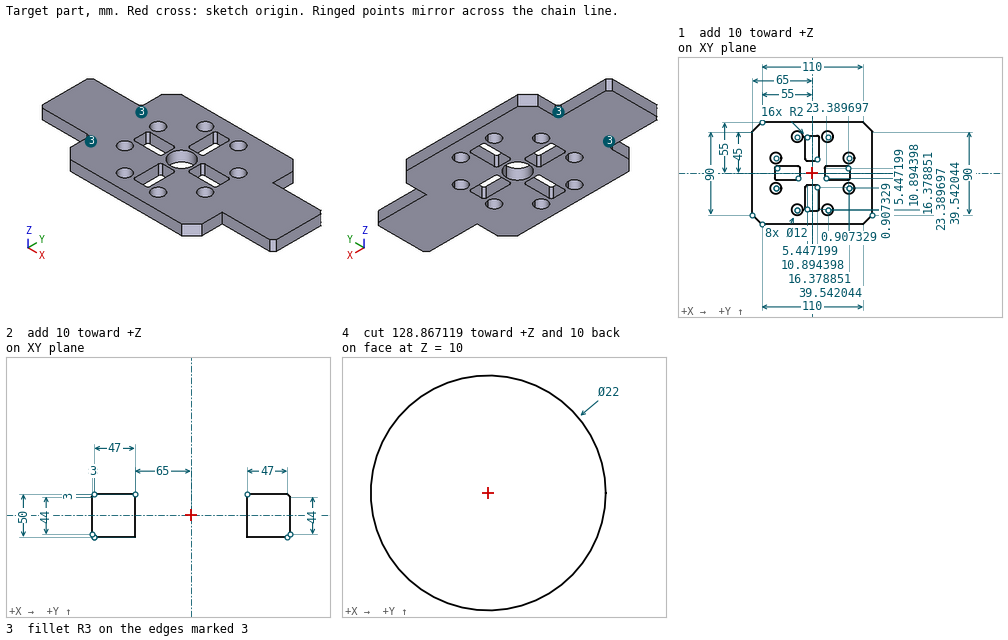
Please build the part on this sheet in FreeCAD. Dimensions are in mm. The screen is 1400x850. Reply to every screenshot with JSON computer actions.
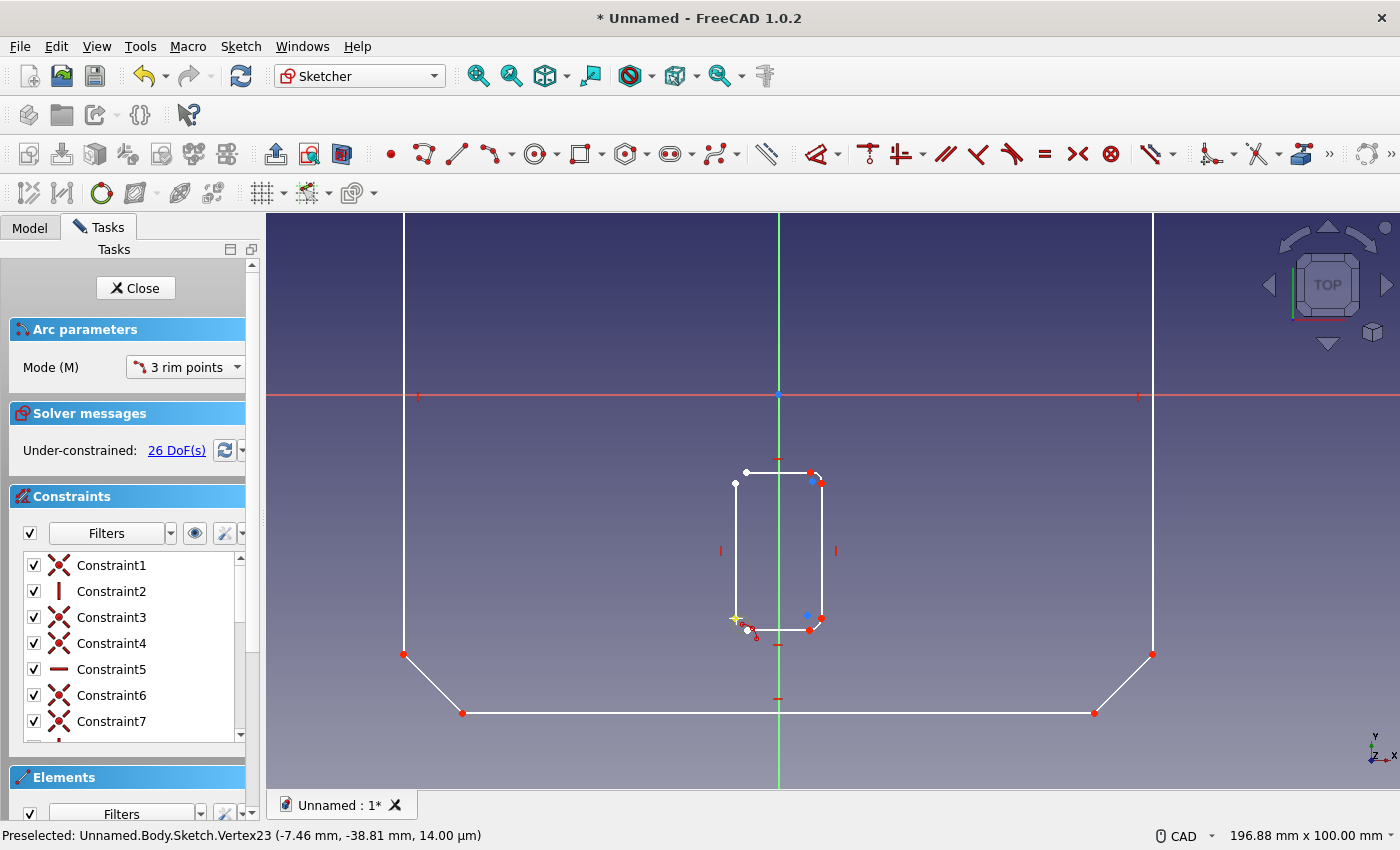
{"action": "scroll", "coordinate": [739, 625], "scroll_direction": "up", "scroll_amount": 8}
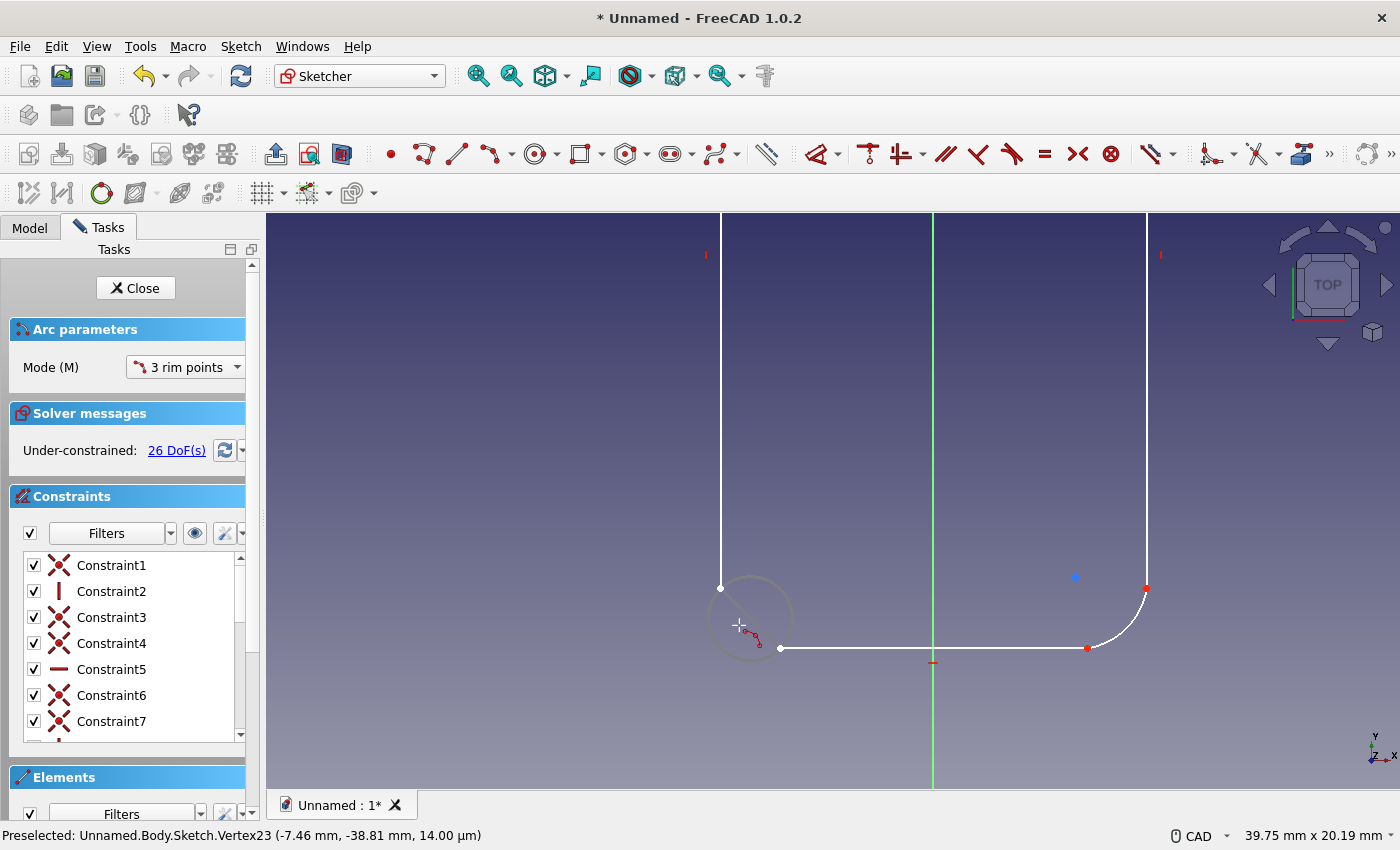
{"action": "left_click", "coordinate": [738, 624]}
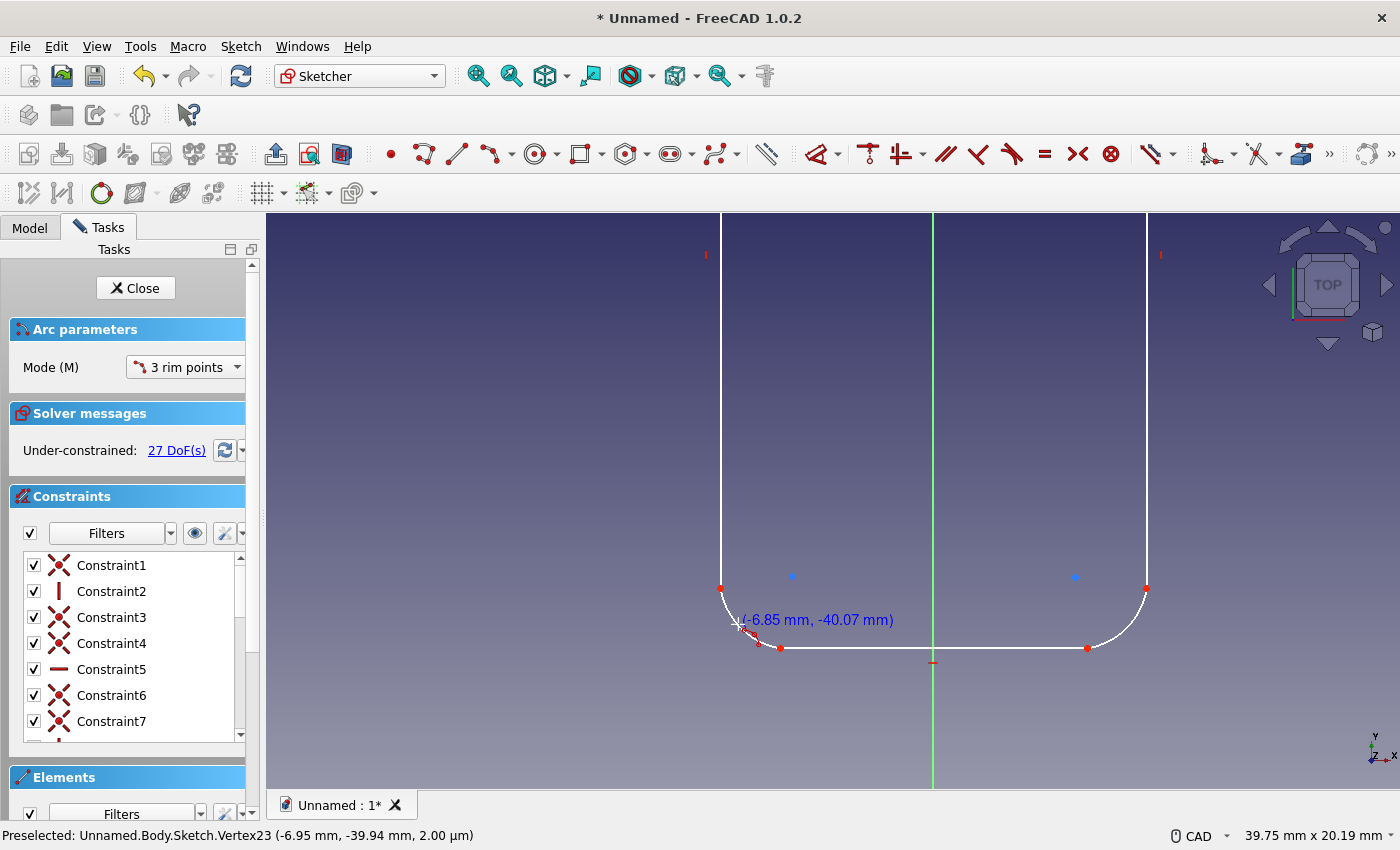
{"action": "scroll", "coordinate": [743, 628], "scroll_direction": "down", "scroll_amount": 11}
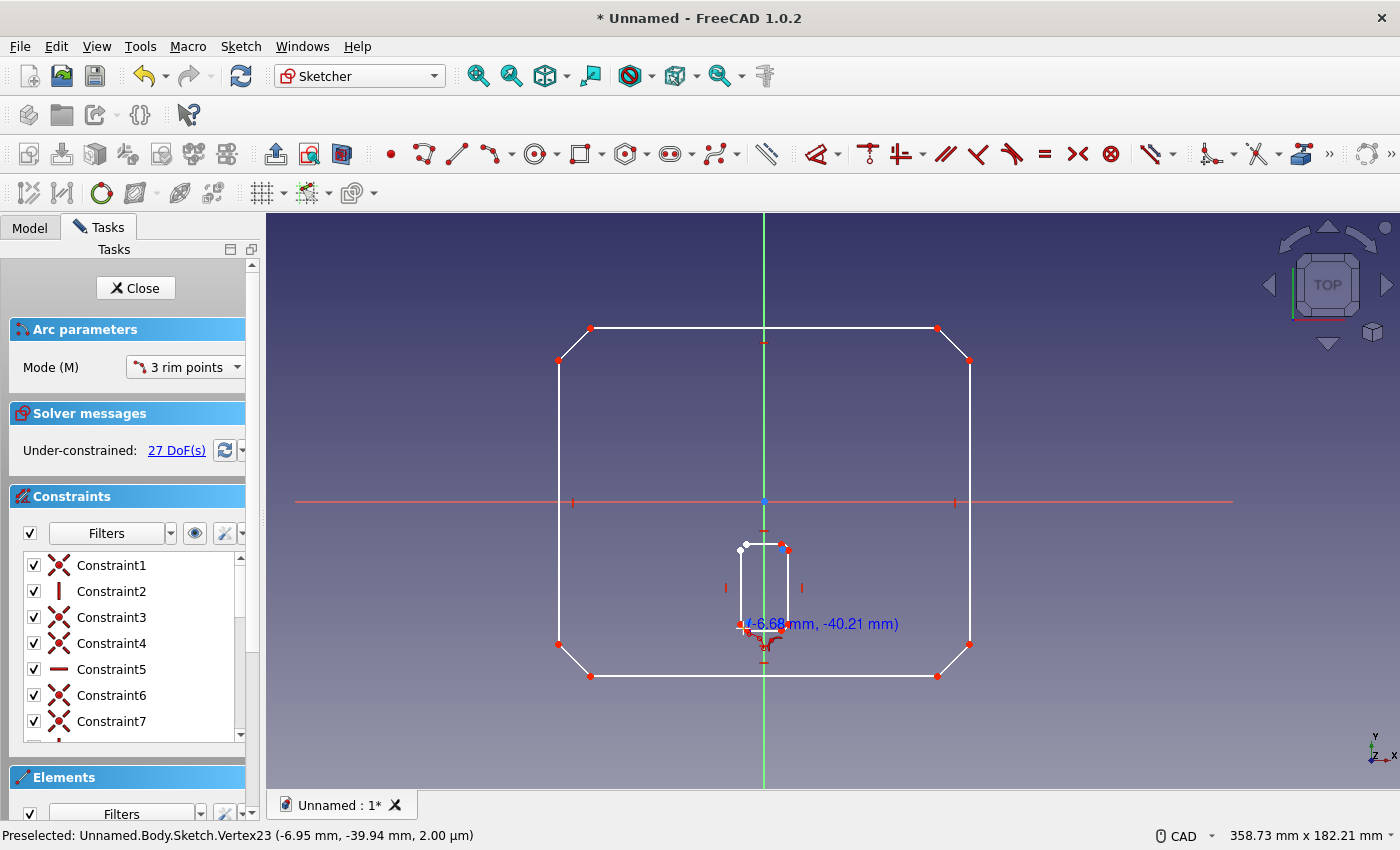
{"action": "scroll", "coordinate": [741, 550], "scroll_direction": "up", "scroll_amount": 3}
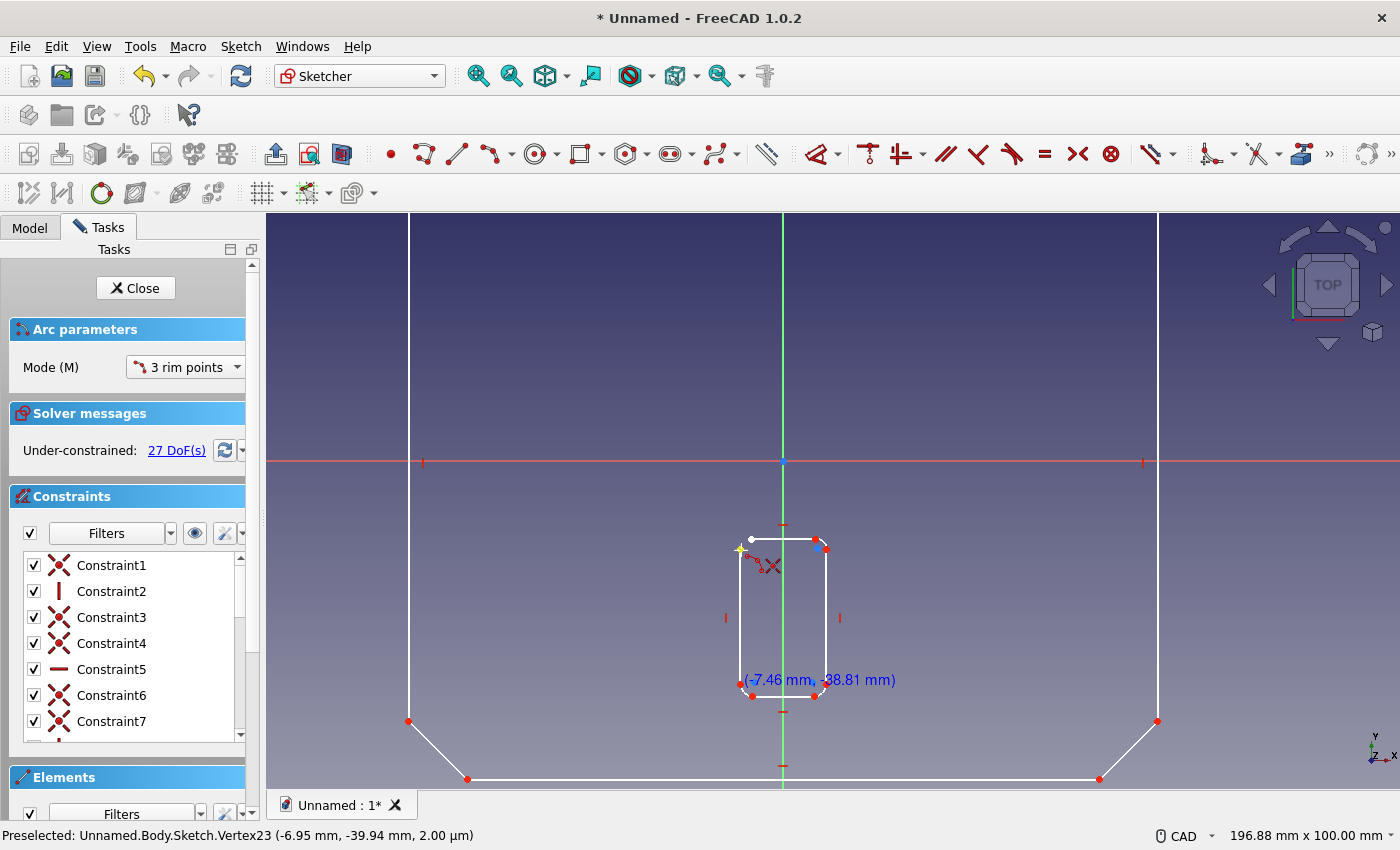
{"action": "left_click", "coordinate": [740, 550]}
{"action": "left_click", "coordinate": [751, 539]}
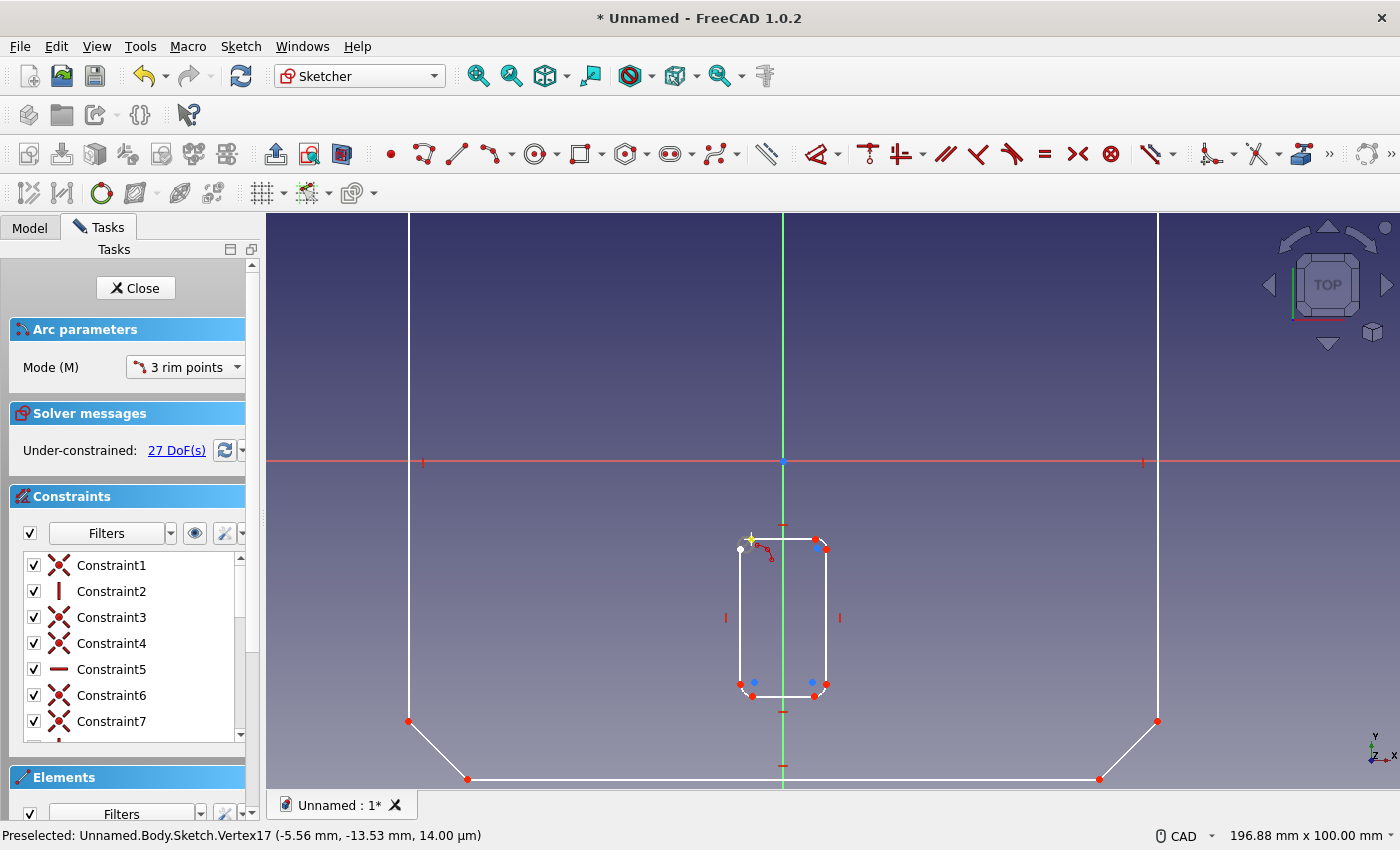
{"action": "scroll", "coordinate": [744, 541], "scroll_direction": "up", "scroll_amount": 8}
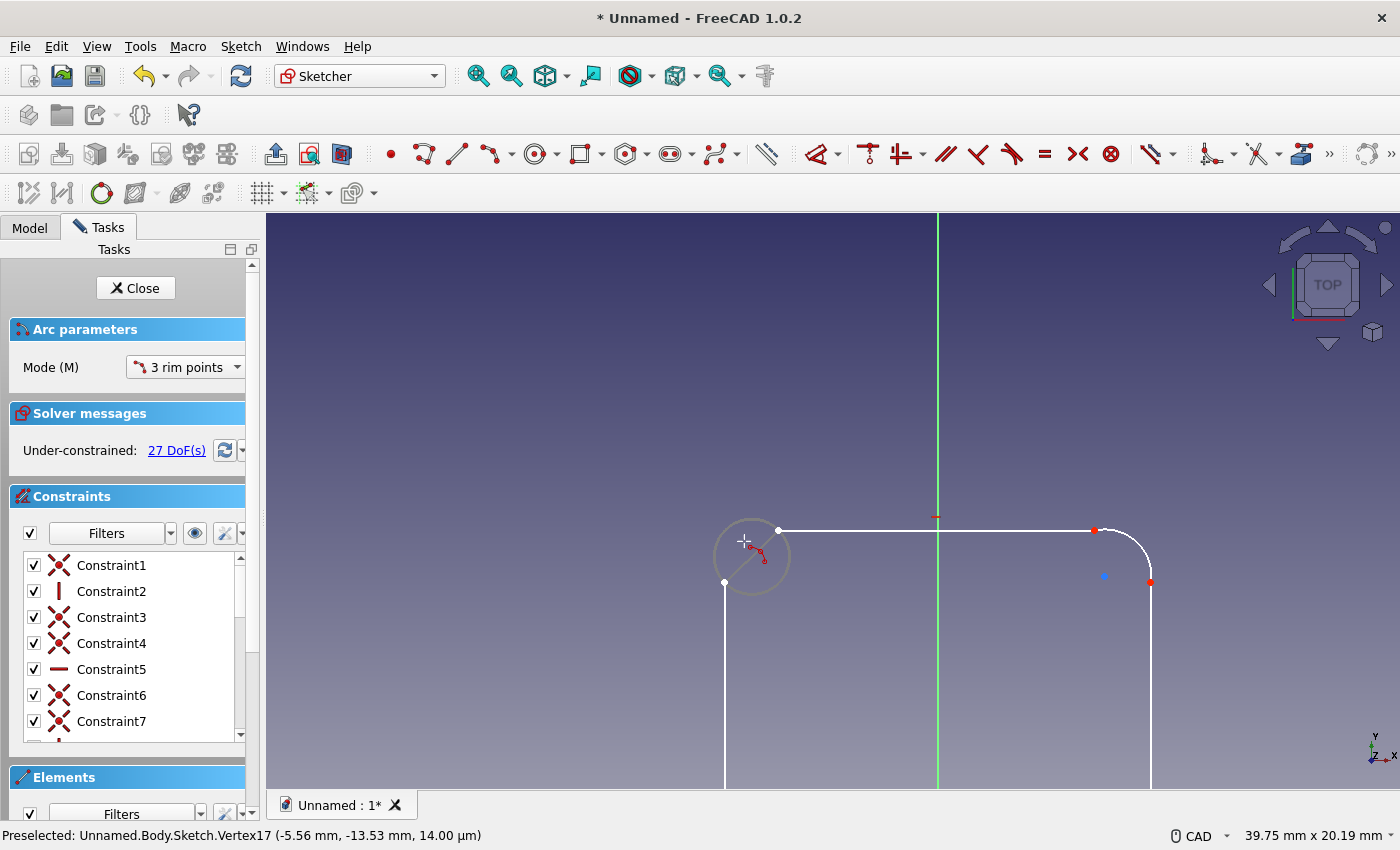
{"action": "left_click", "coordinate": [742, 539]}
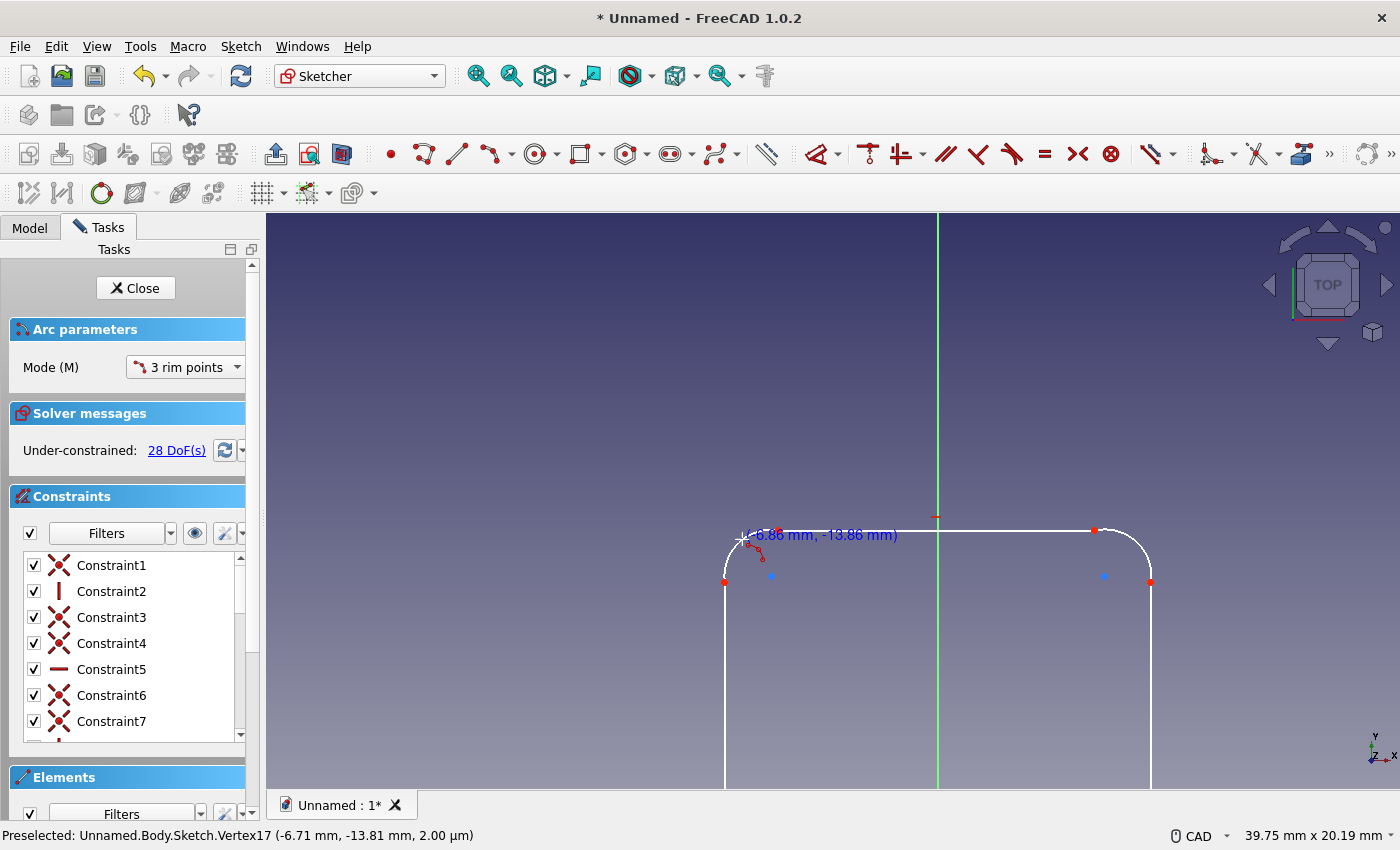
{"action": "left_click", "coordinate": [457, 154]}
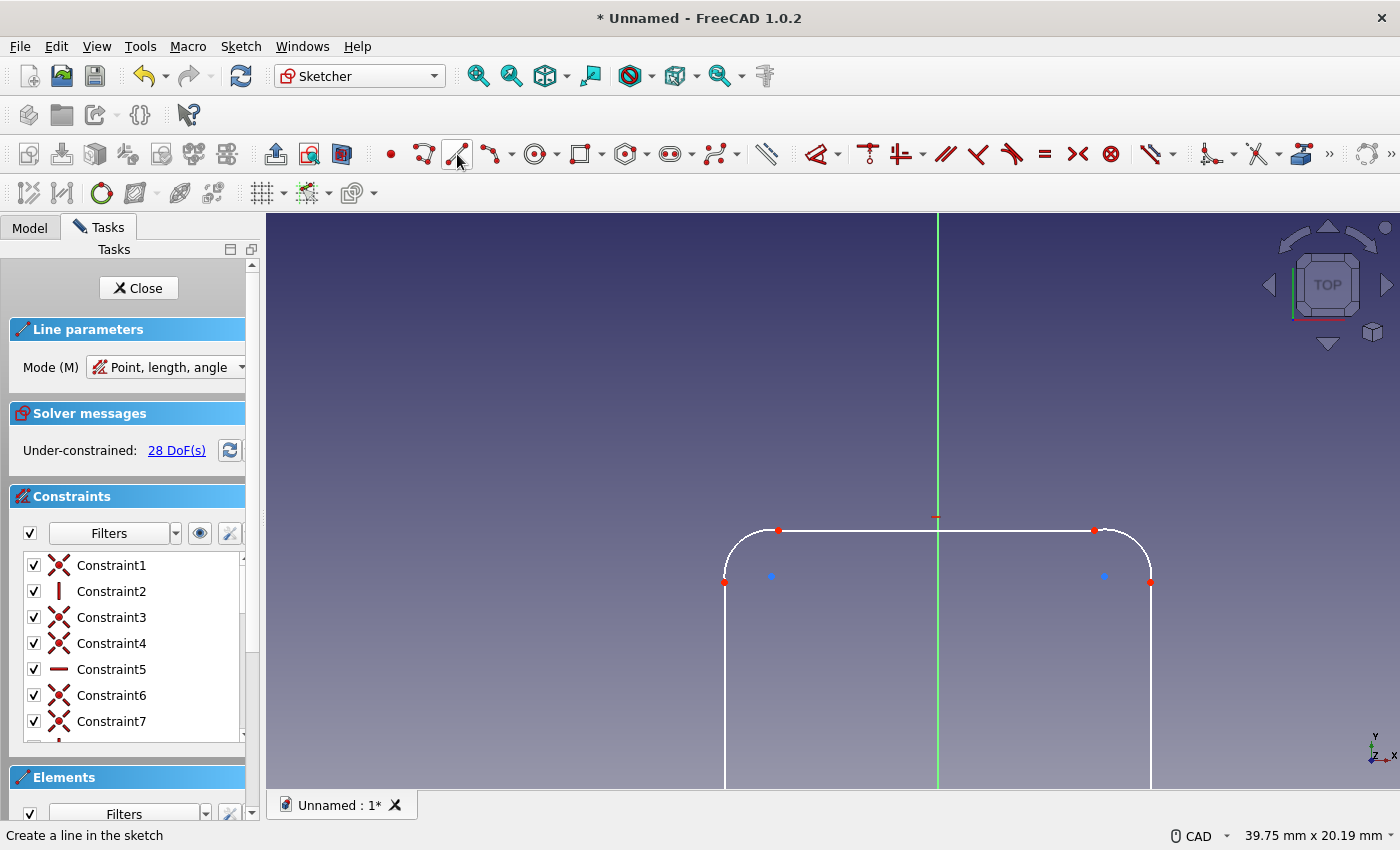
{"action": "scroll", "coordinate": [743, 545], "scroll_direction": "down", "scroll_amount": 11}